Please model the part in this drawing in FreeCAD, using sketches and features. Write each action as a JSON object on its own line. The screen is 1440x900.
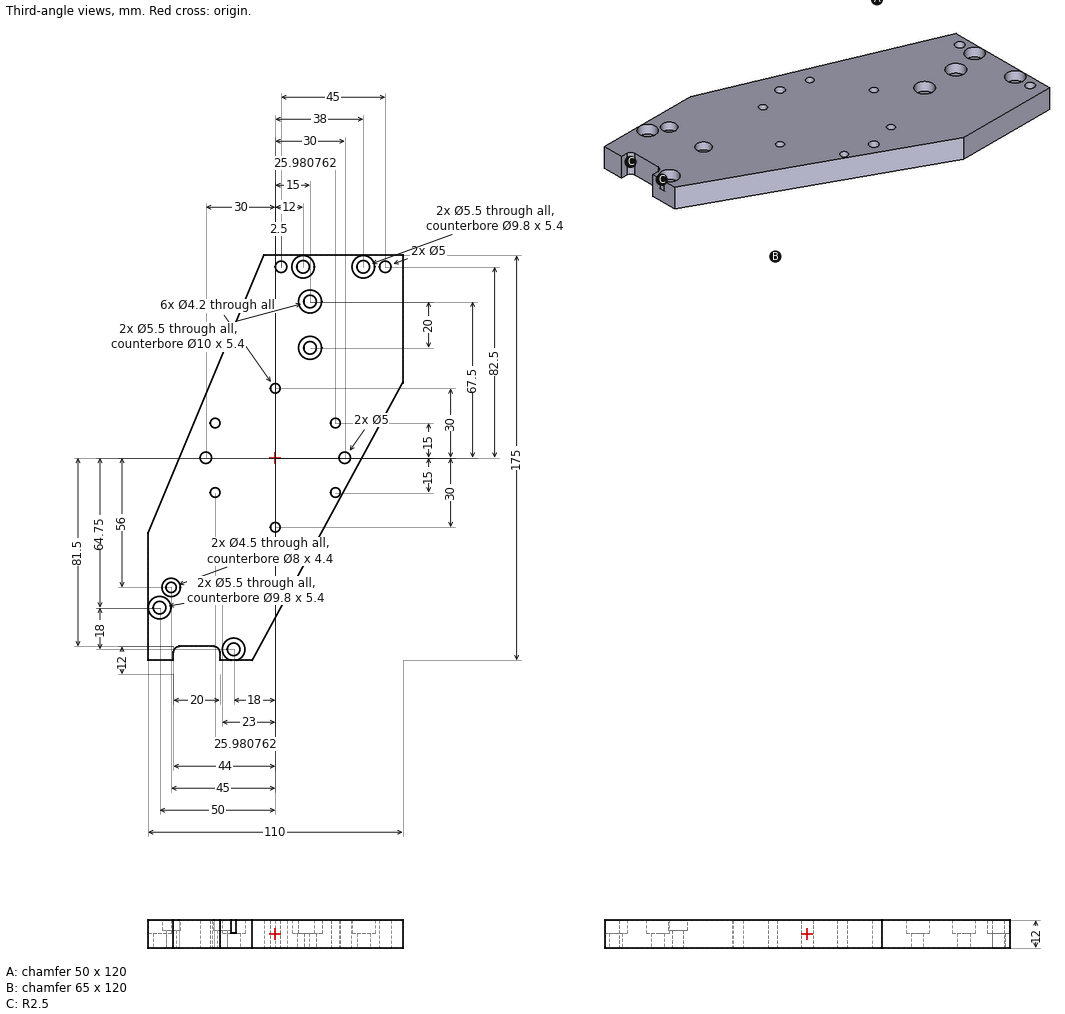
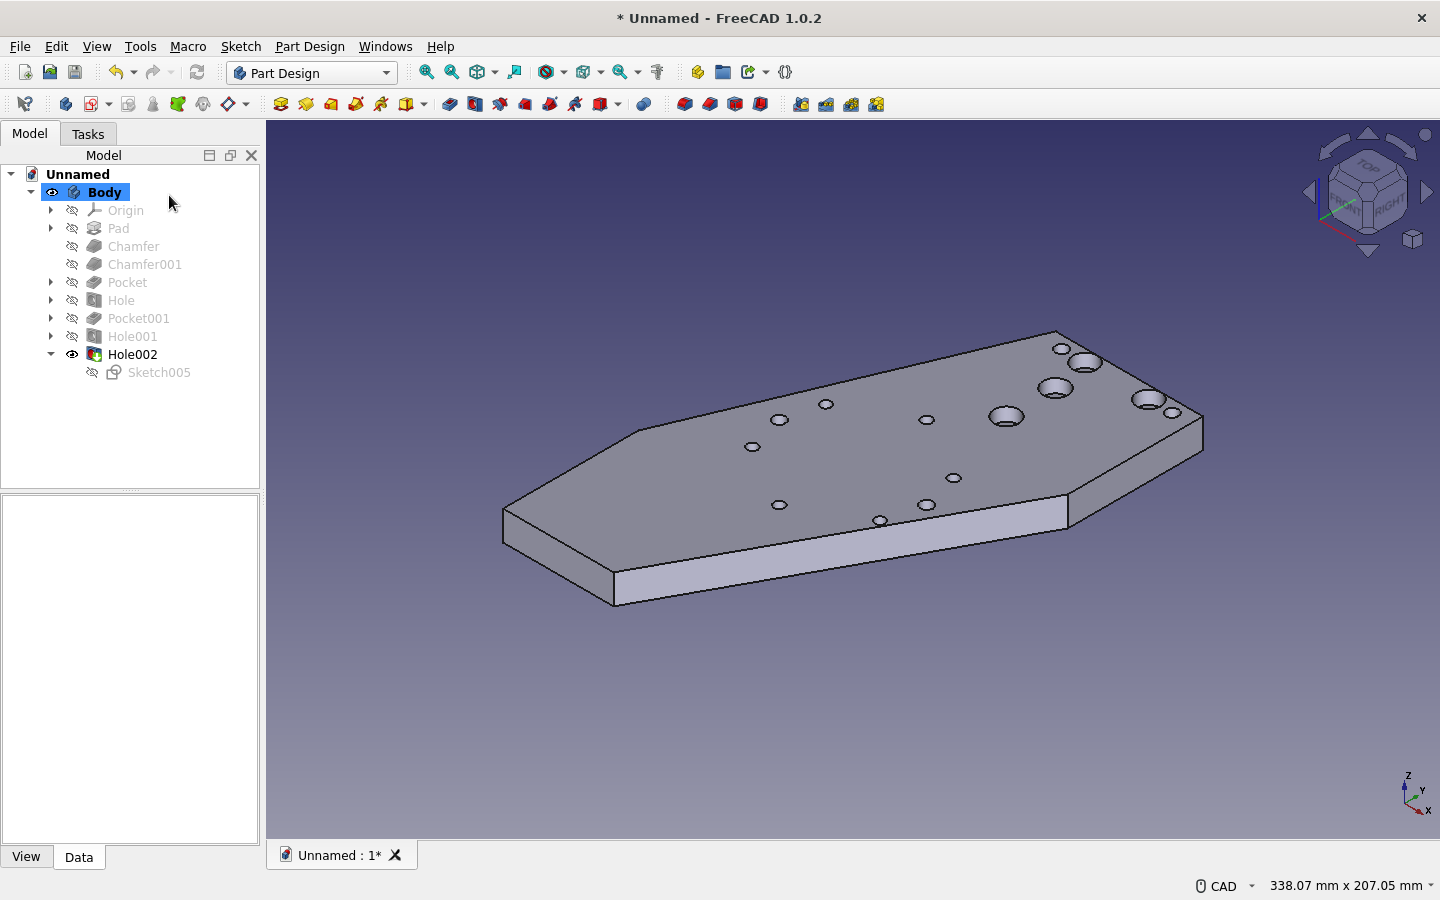
{"action": "left_click", "coordinate": [853, 461]}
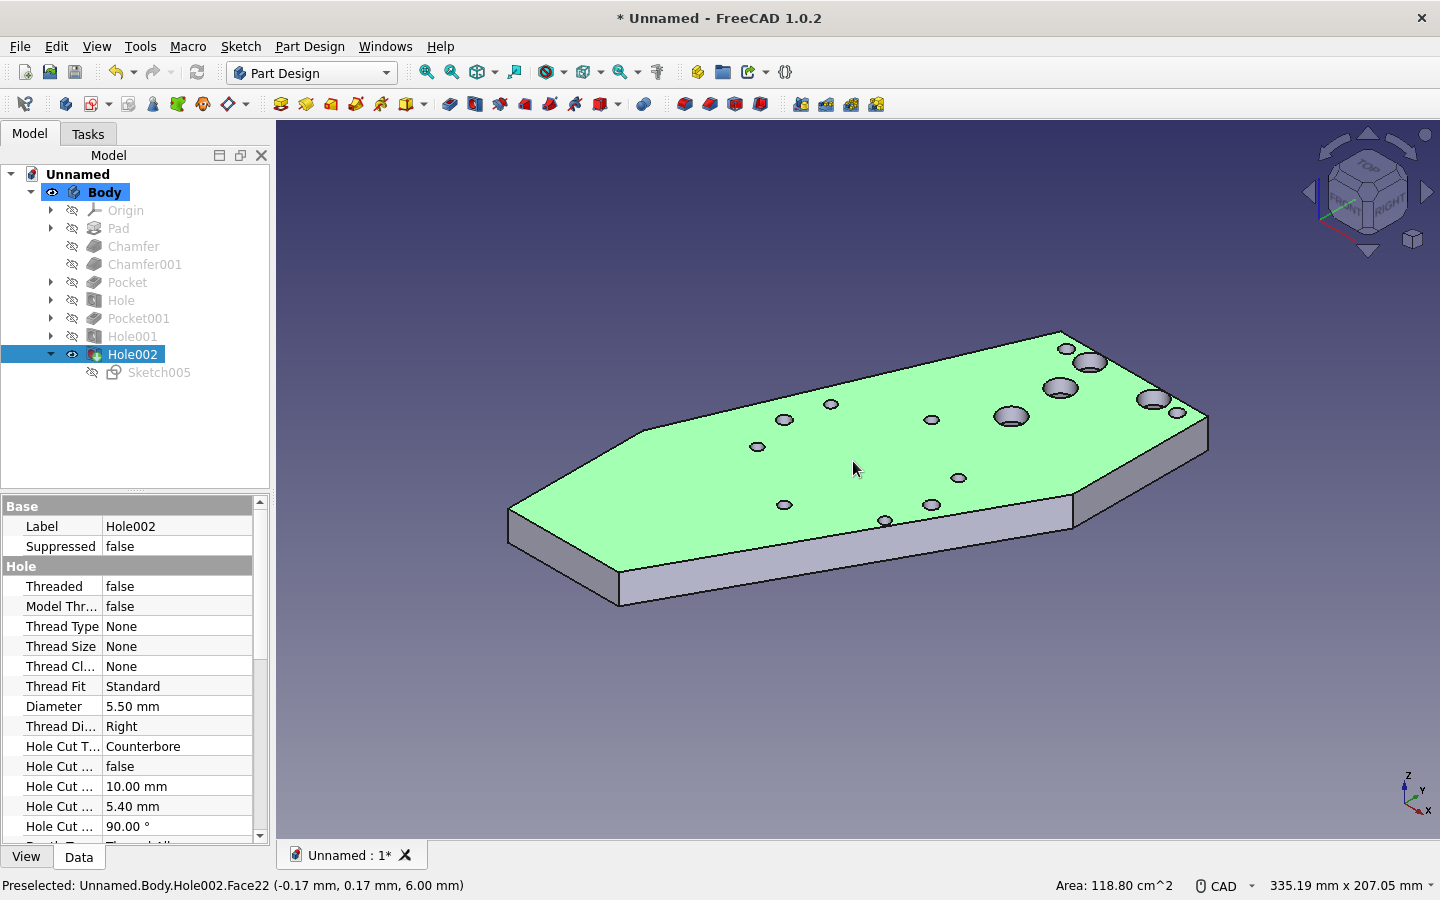
{"action": "left_click", "coordinate": [90, 104]}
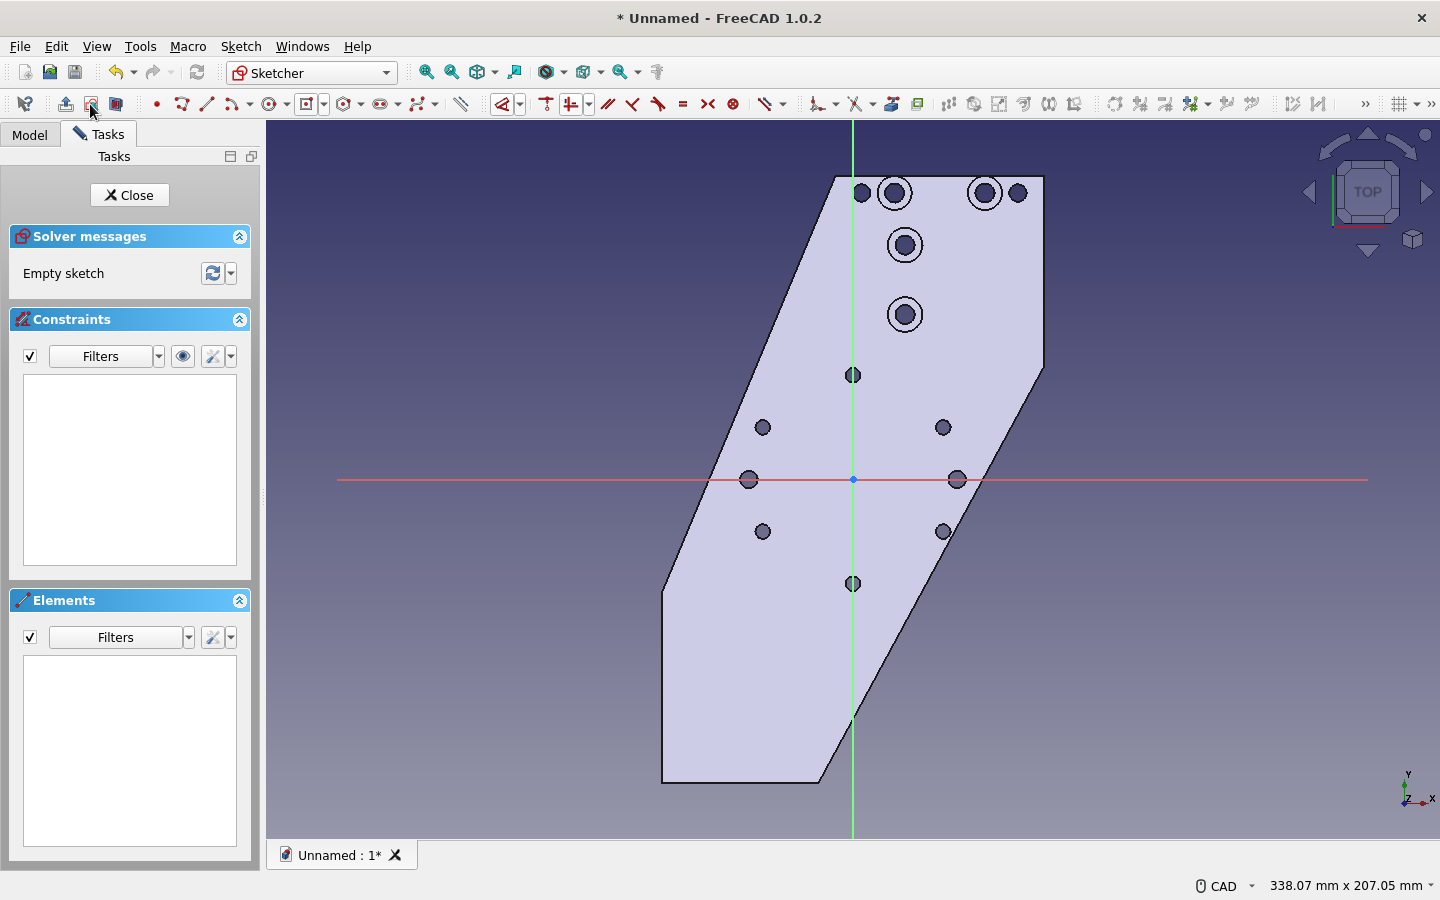
{"action": "scroll", "coordinate": [760, 663], "scroll_direction": "up", "scroll_amount": 4}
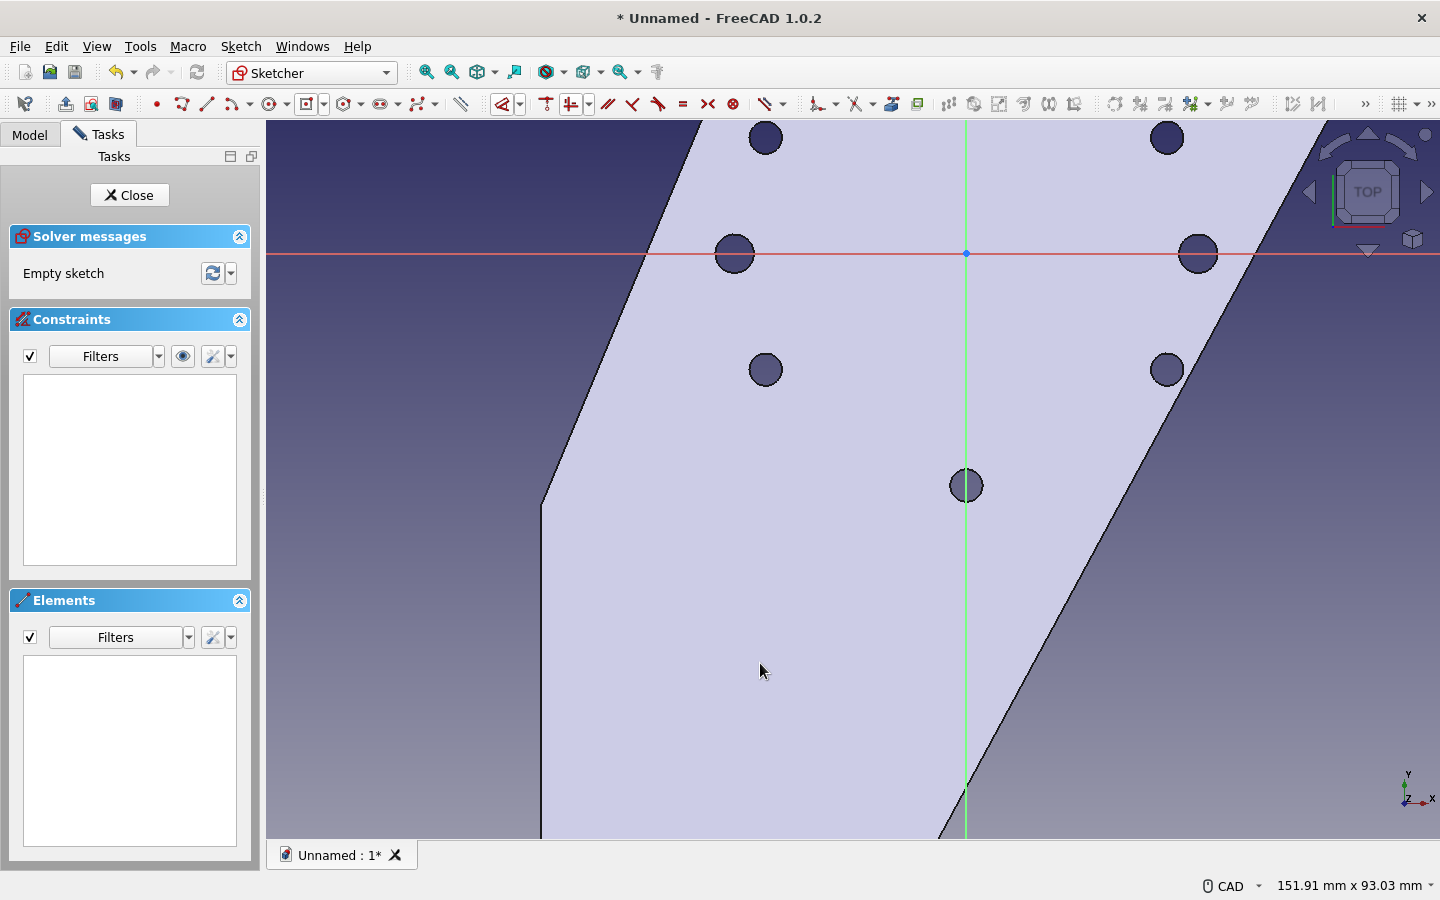
{"action": "key", "text": "g c"}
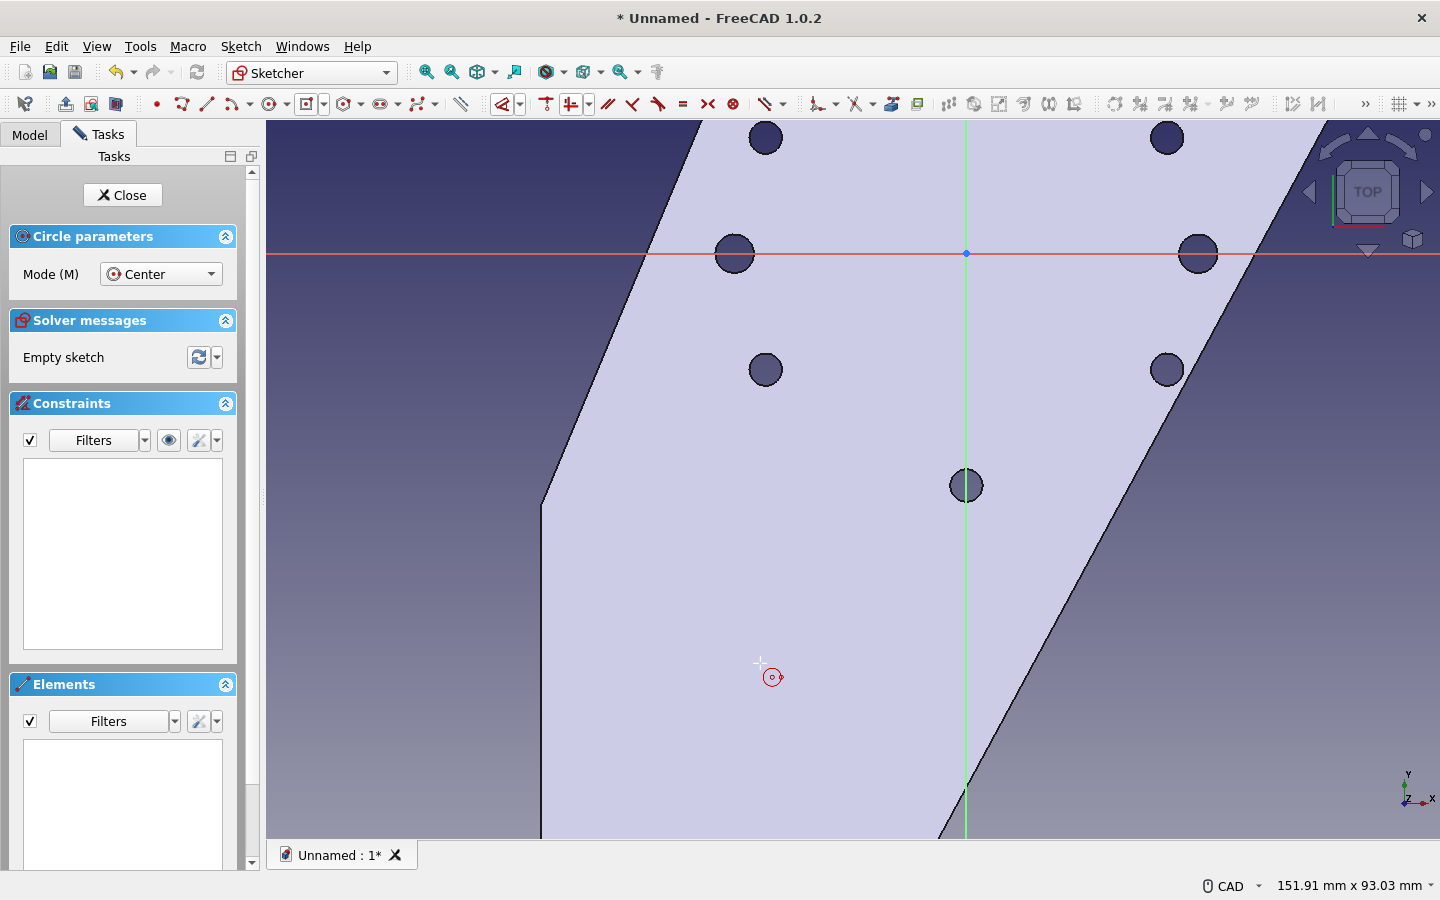
{"action": "scroll", "coordinate": [619, 686], "scroll_direction": "up", "scroll_amount": 2}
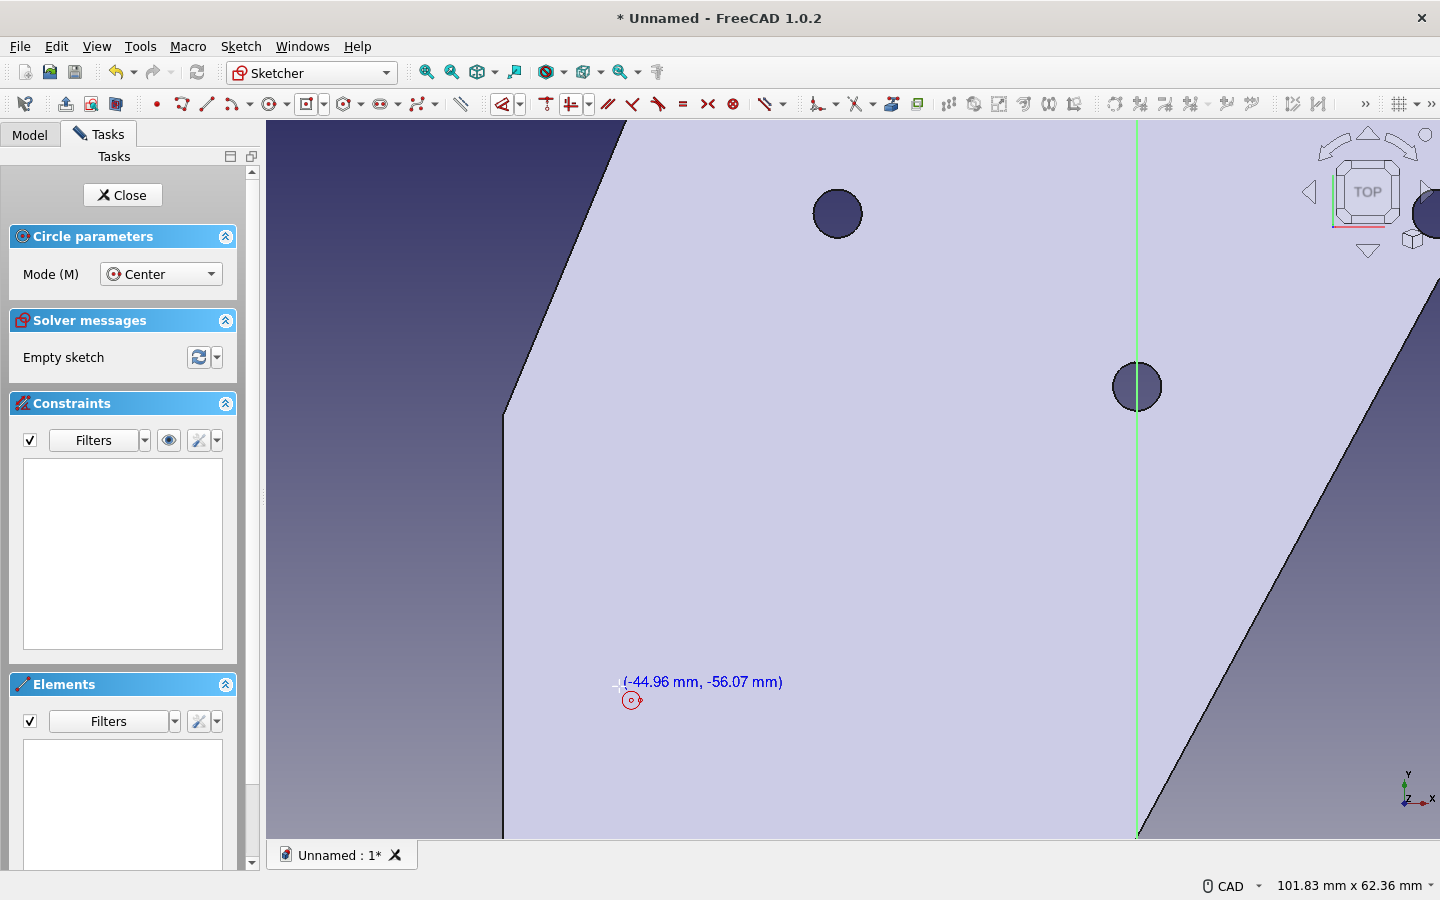
{"action": "left_click", "coordinate": [618, 686]}
{"action": "left_click", "coordinate": [637, 668]}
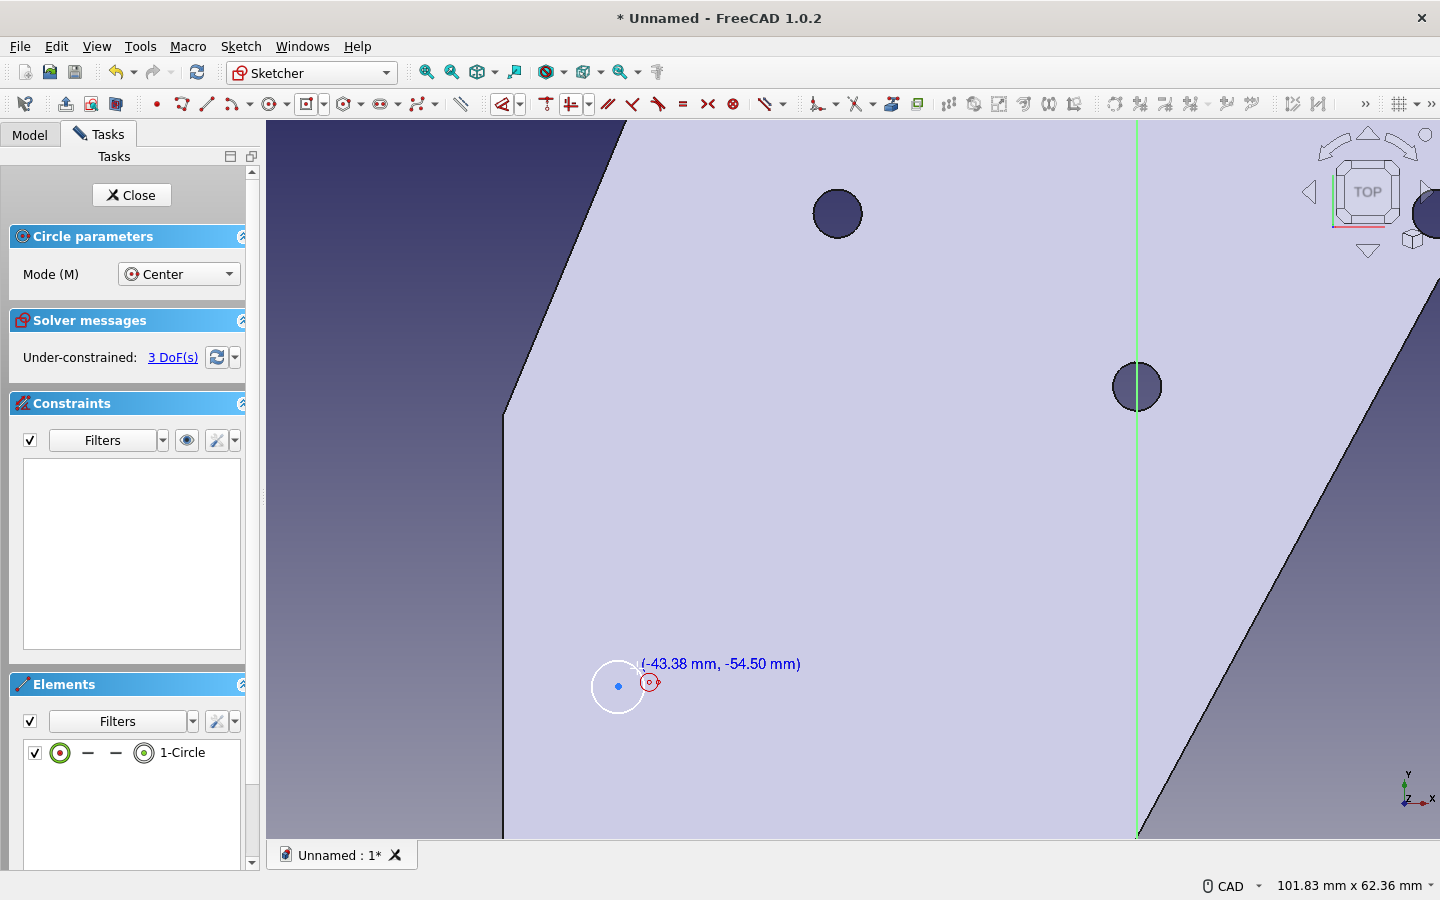
{"action": "left_click", "coordinate": [872, 686]}
{"action": "left_click", "coordinate": [890, 668]}
{"action": "key", "text": "Escape"}